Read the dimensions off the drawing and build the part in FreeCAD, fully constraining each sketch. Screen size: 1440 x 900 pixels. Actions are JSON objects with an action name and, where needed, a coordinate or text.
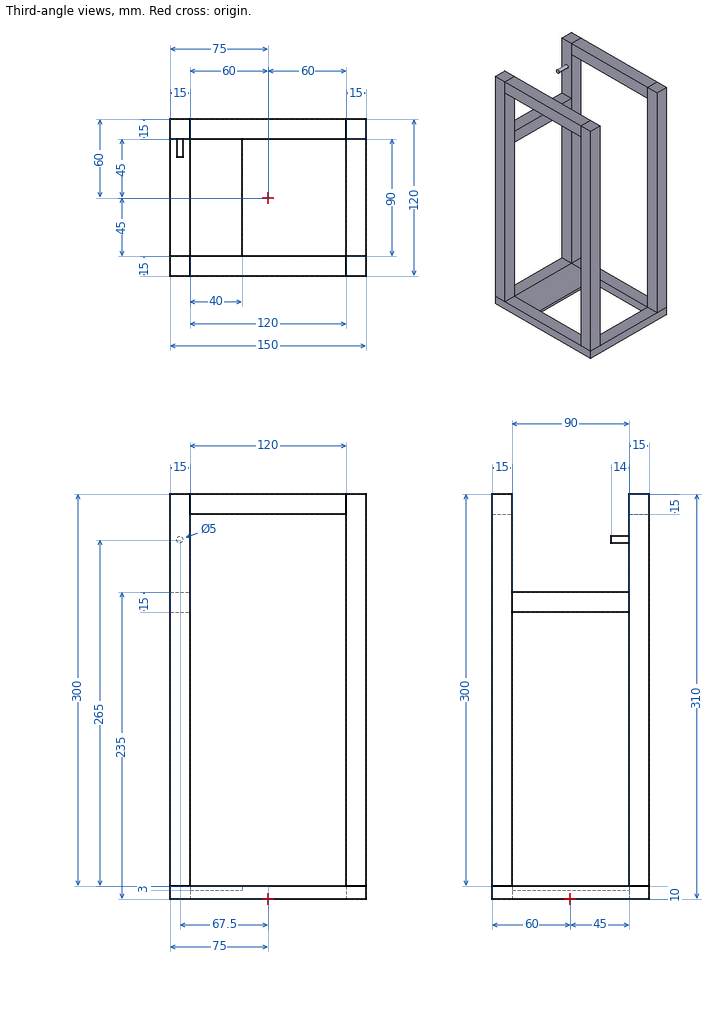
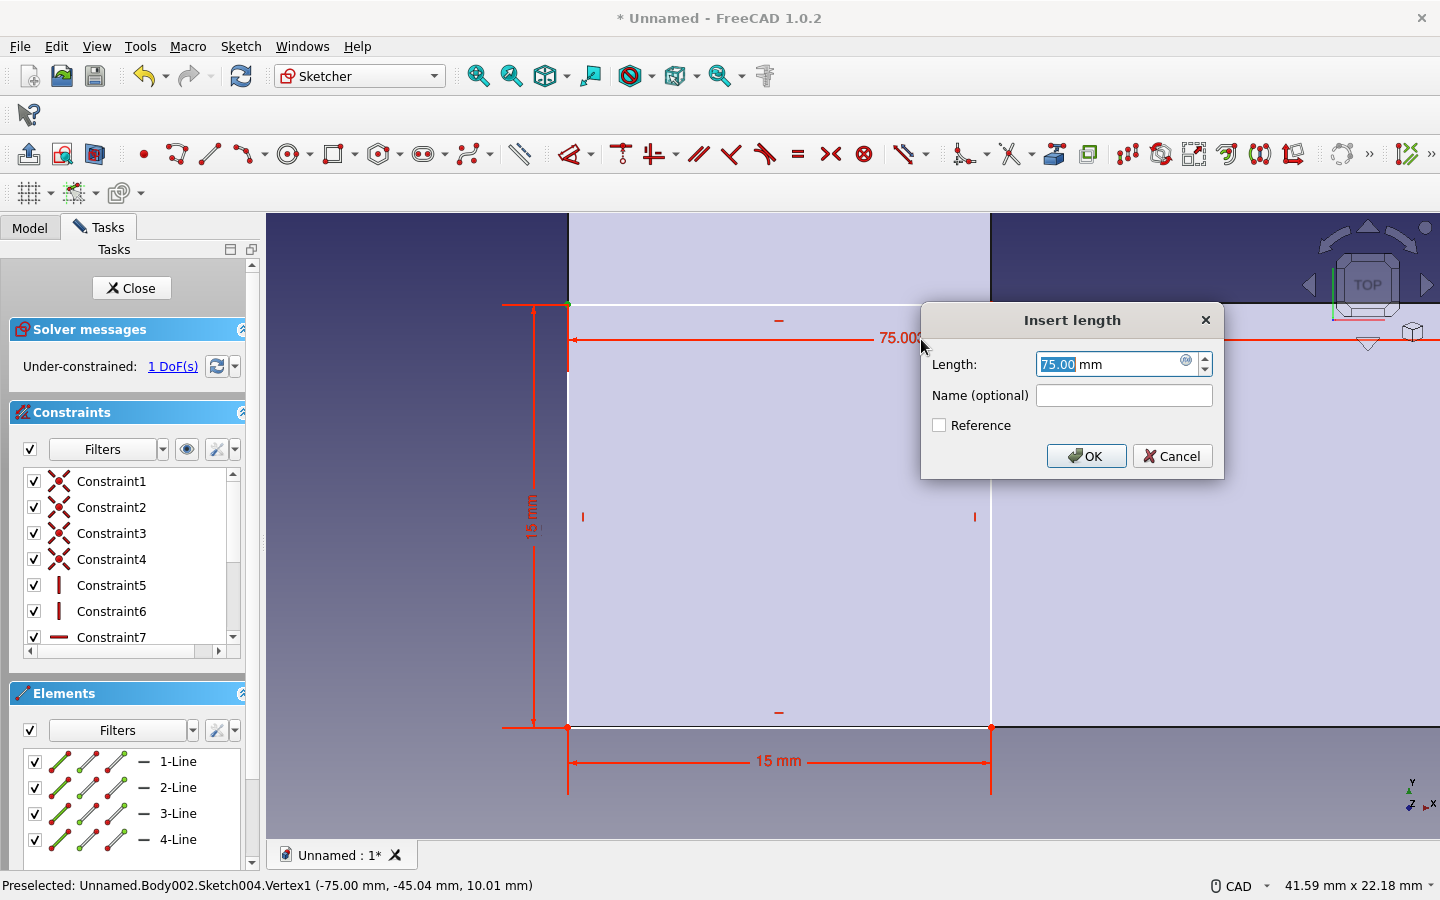
{"action": "type", "text": "75"}
{"action": "key", "text": "Return"}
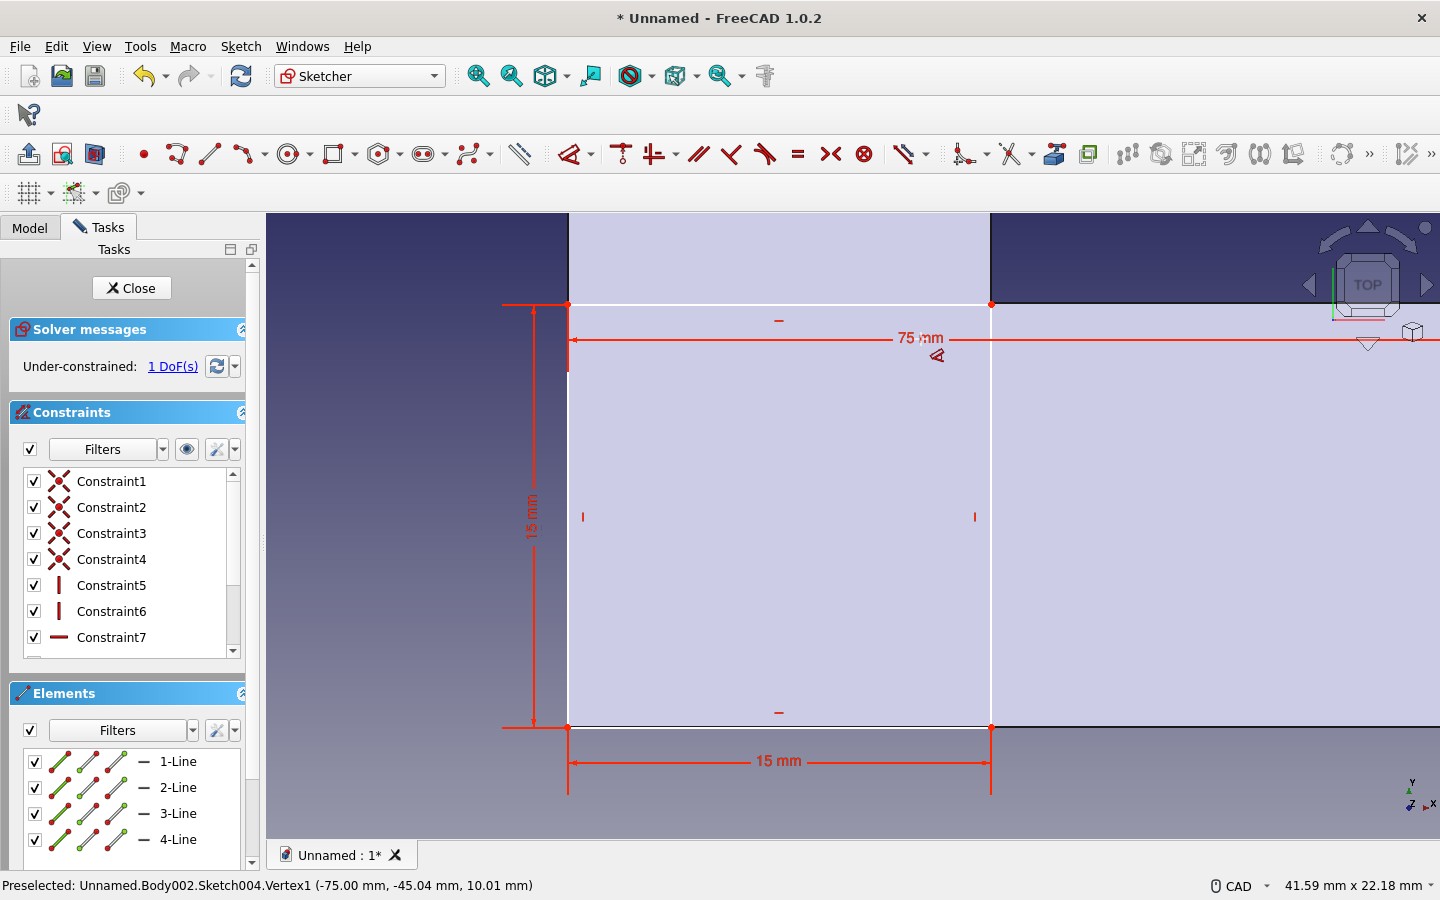
{"action": "left_click", "coordinate": [568, 305]}
{"action": "left_click", "coordinate": [534, 273]}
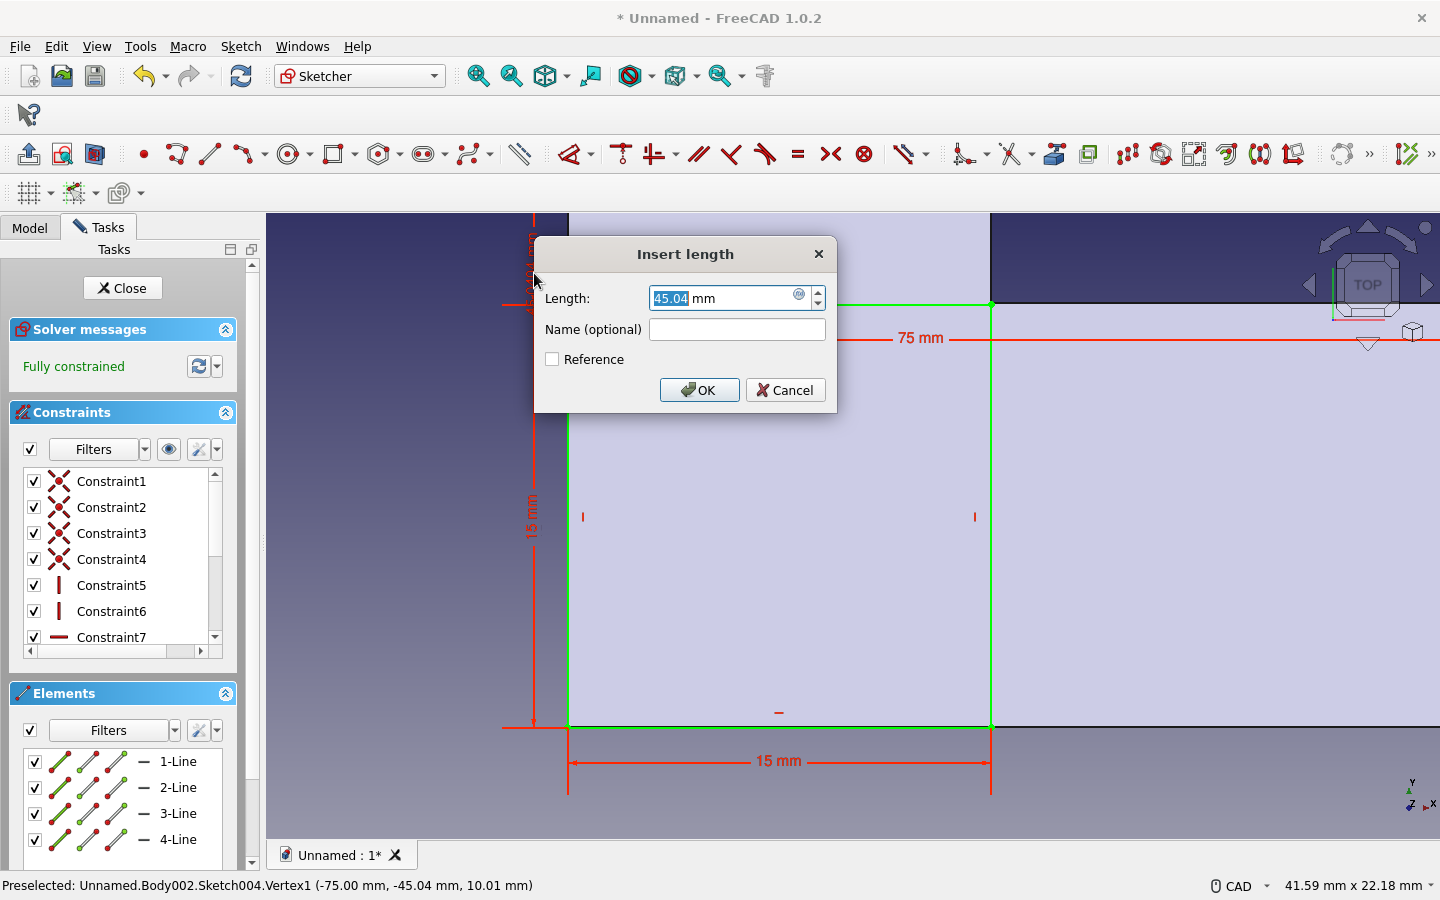
{"action": "type", "text": "45"}
{"action": "key", "text": "Return"}
{"action": "key", "text": "Escape"}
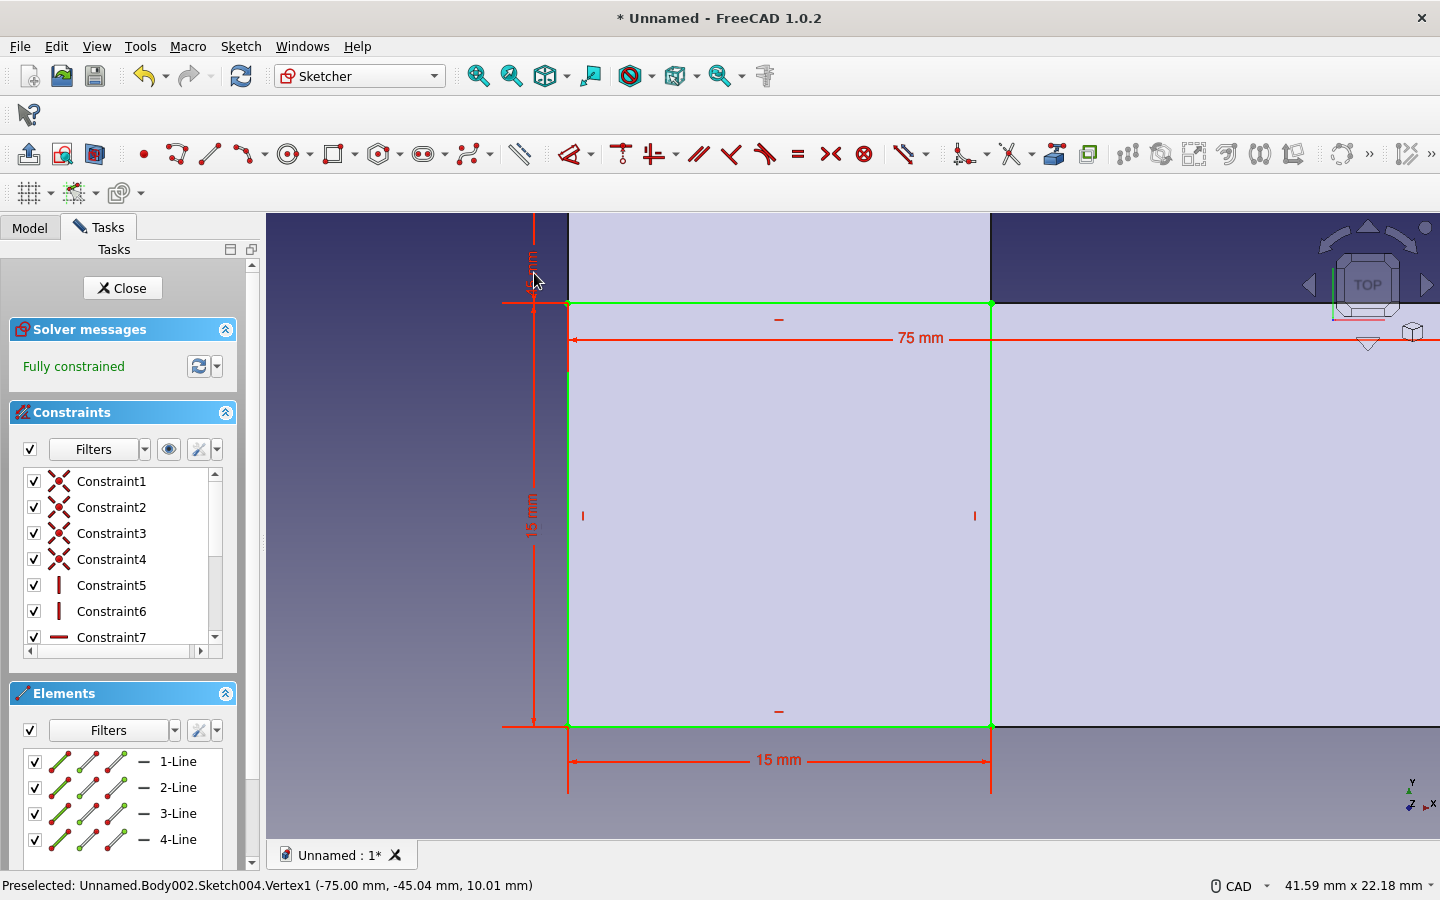
{"action": "left_click", "coordinate": [123, 288]}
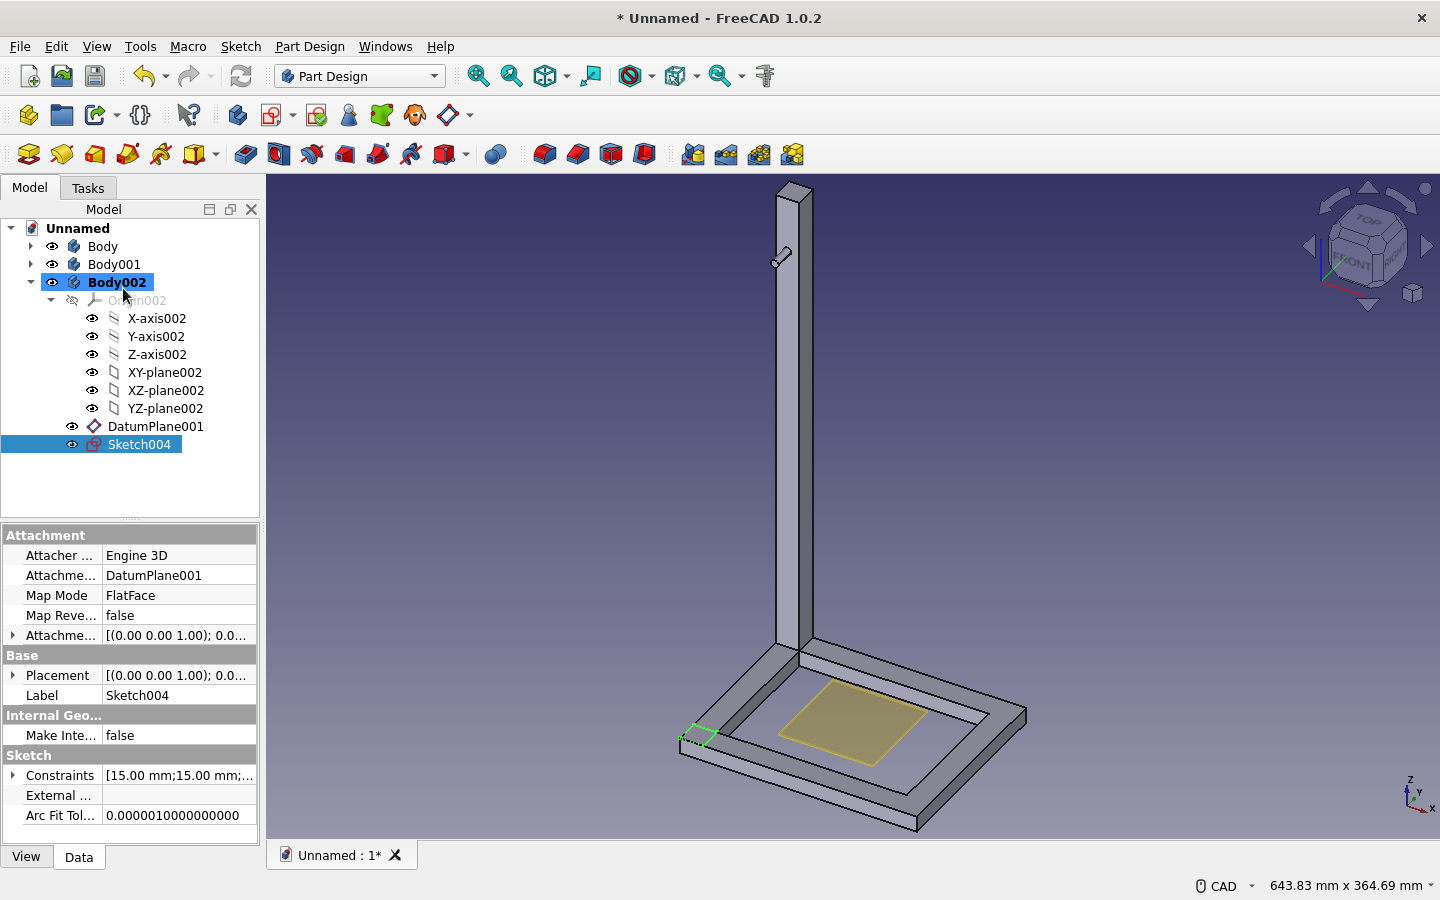
{"action": "left_click", "coordinate": [29, 154]}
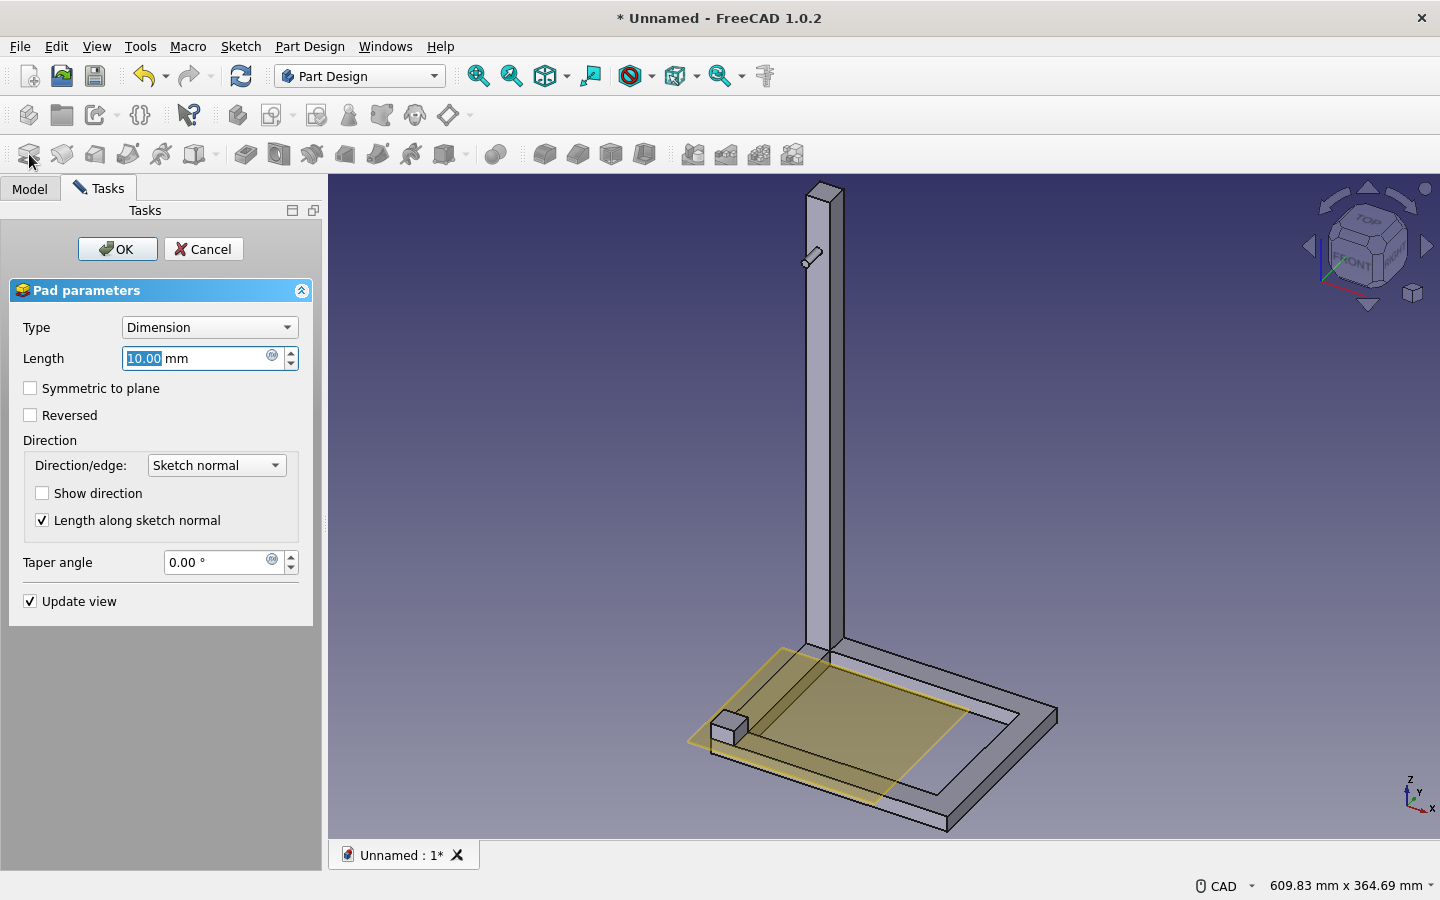
{"action": "type", "text": "300"}
{"action": "key", "text": "Tab"}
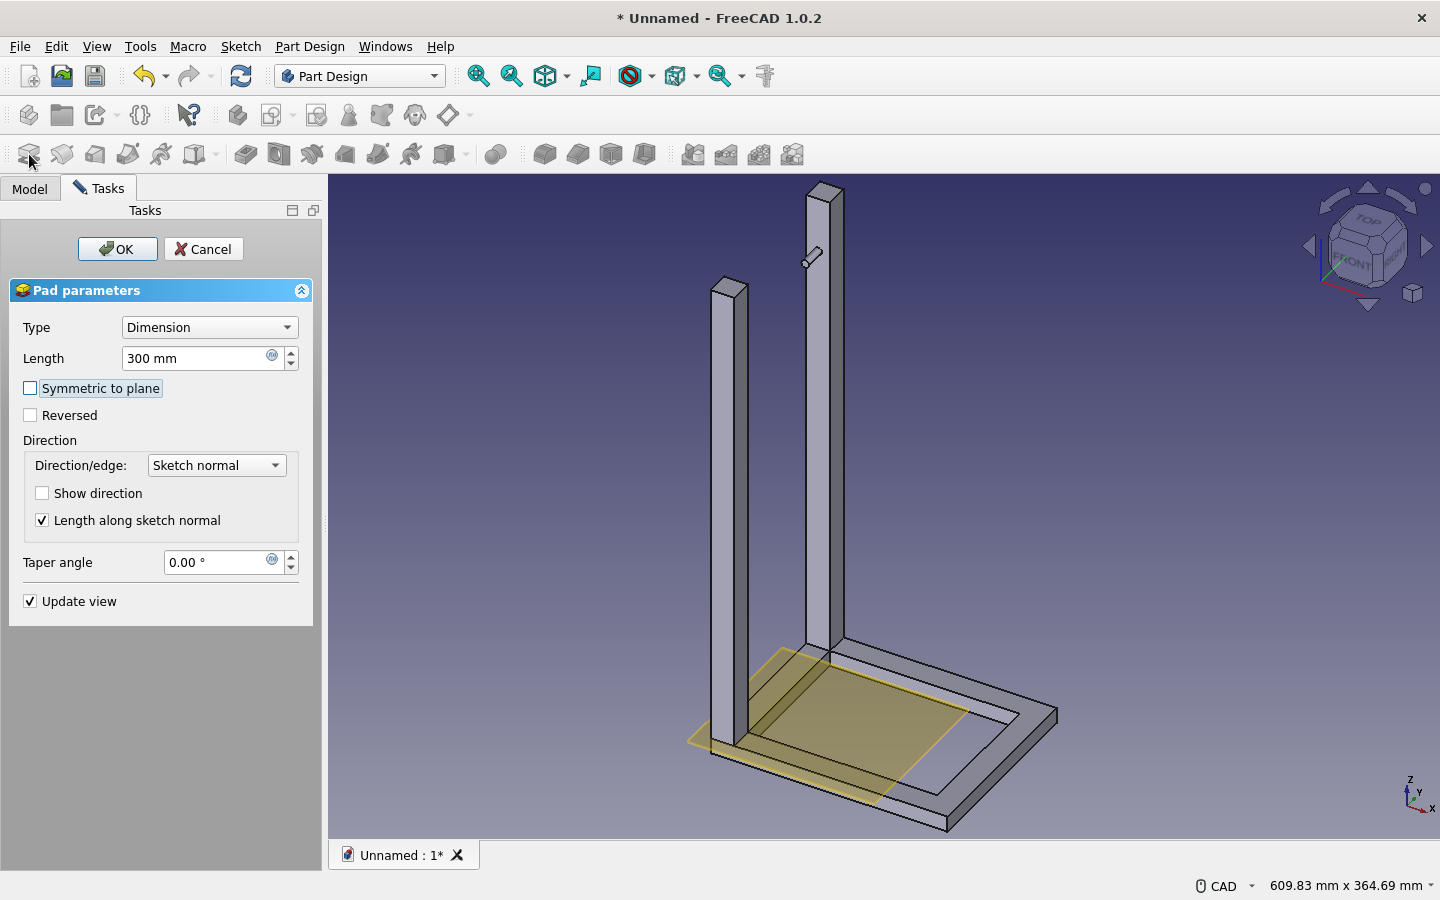
{"action": "left_click", "coordinate": [118, 249]}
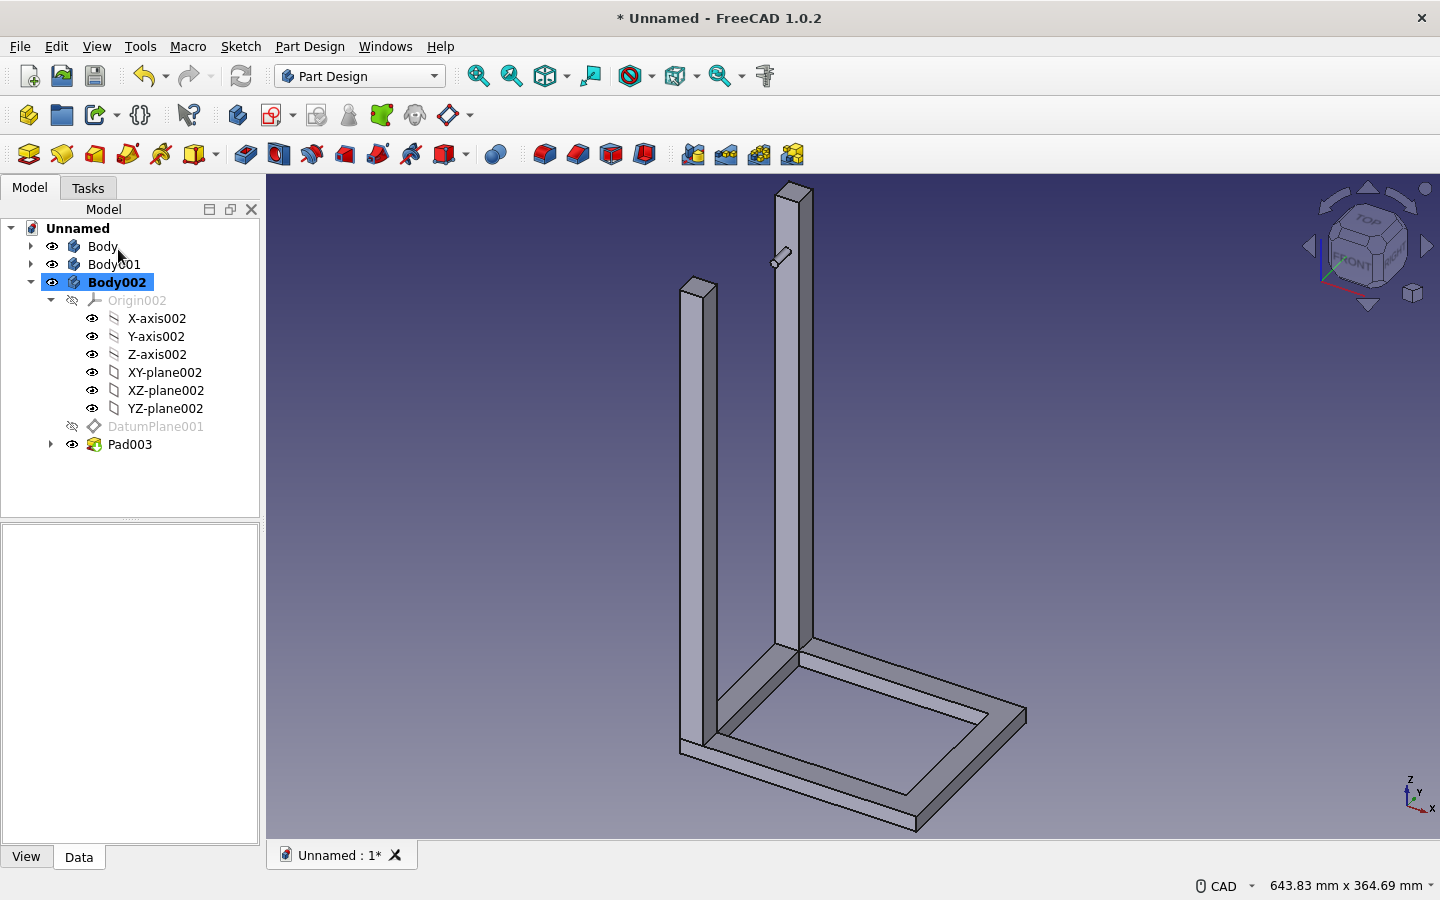
{"action": "left_click", "coordinate": [238, 116]}